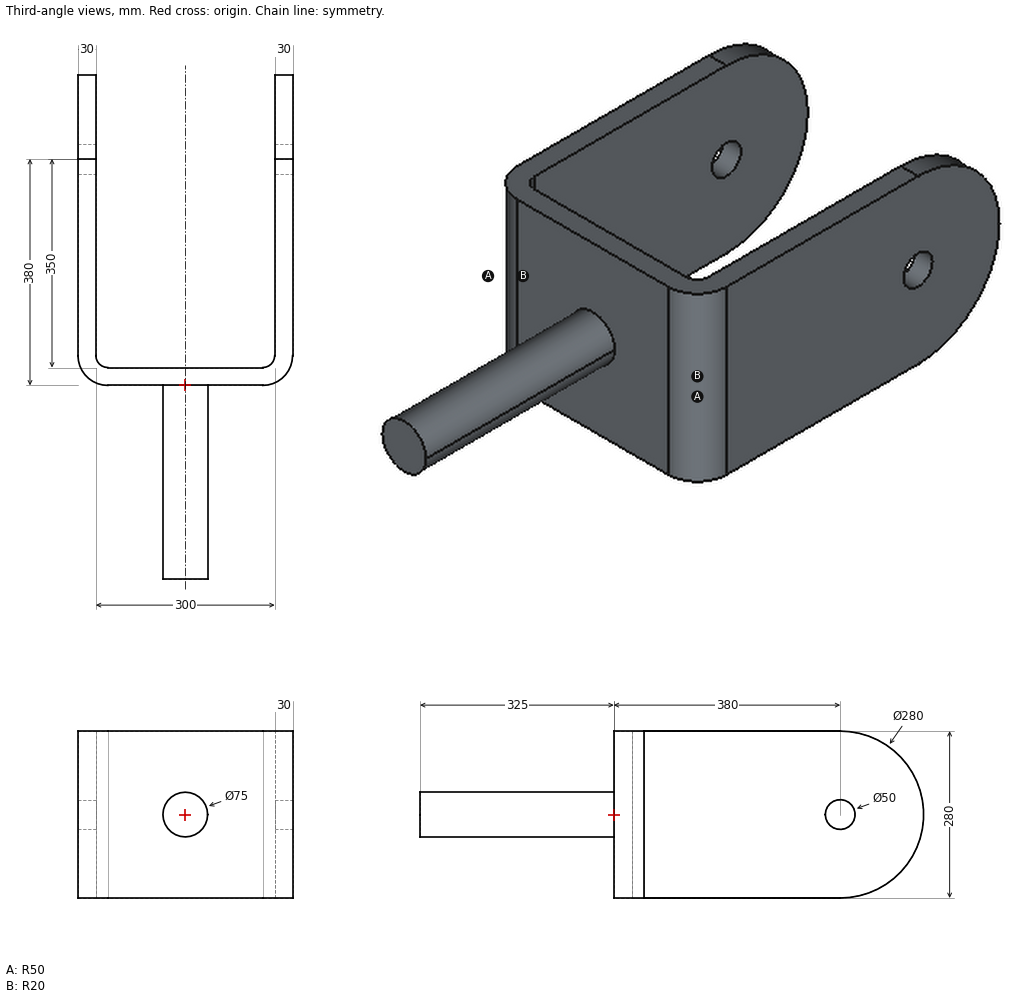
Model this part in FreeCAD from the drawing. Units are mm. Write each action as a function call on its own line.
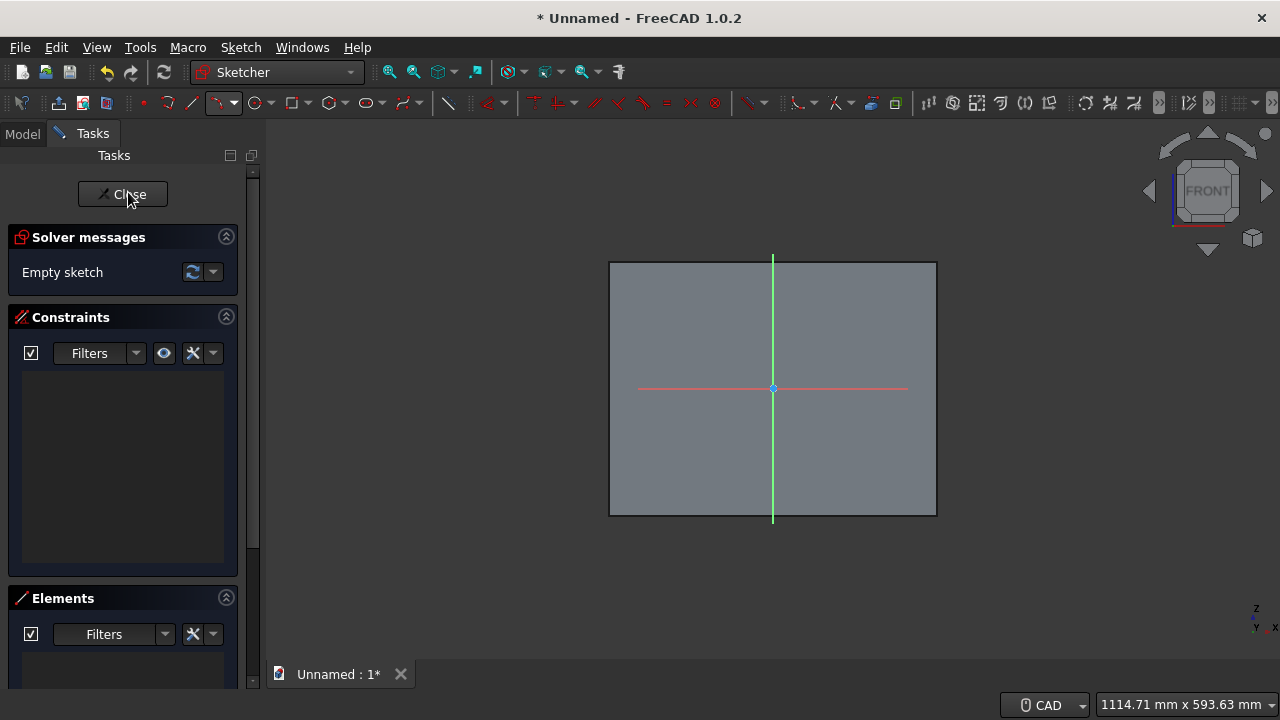
scroll(790, 389, up, 8)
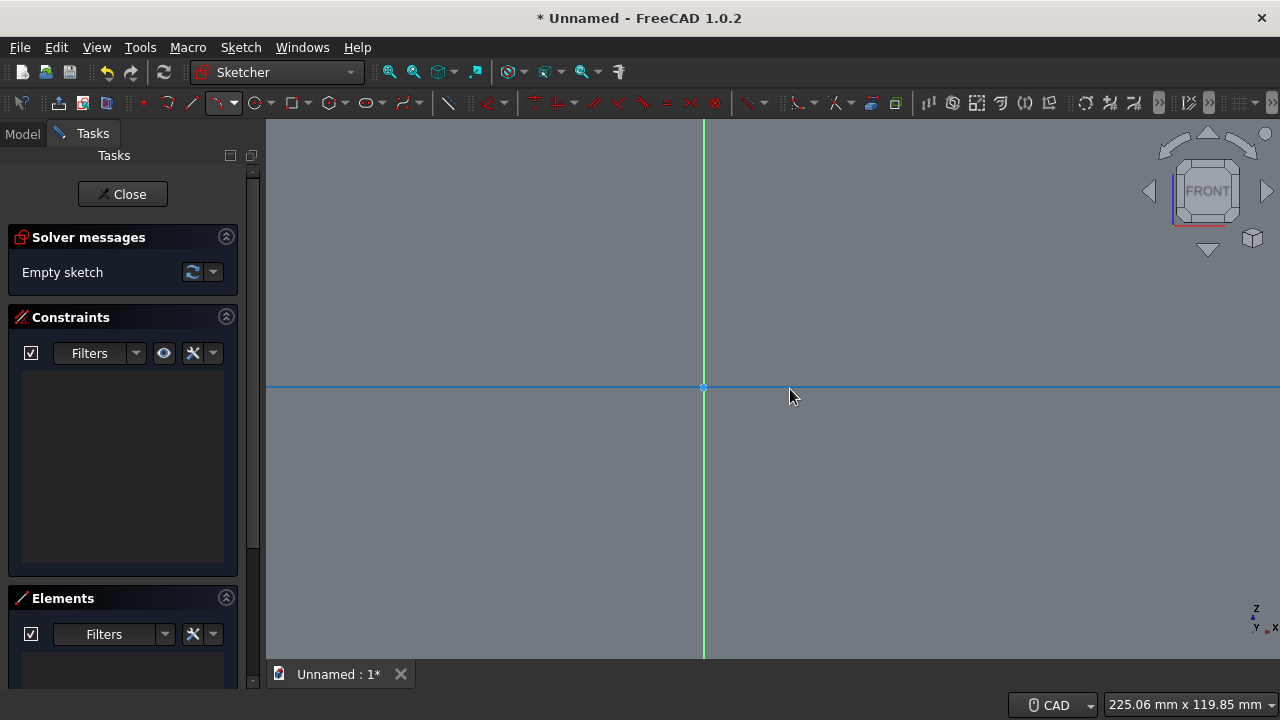
click(256, 104)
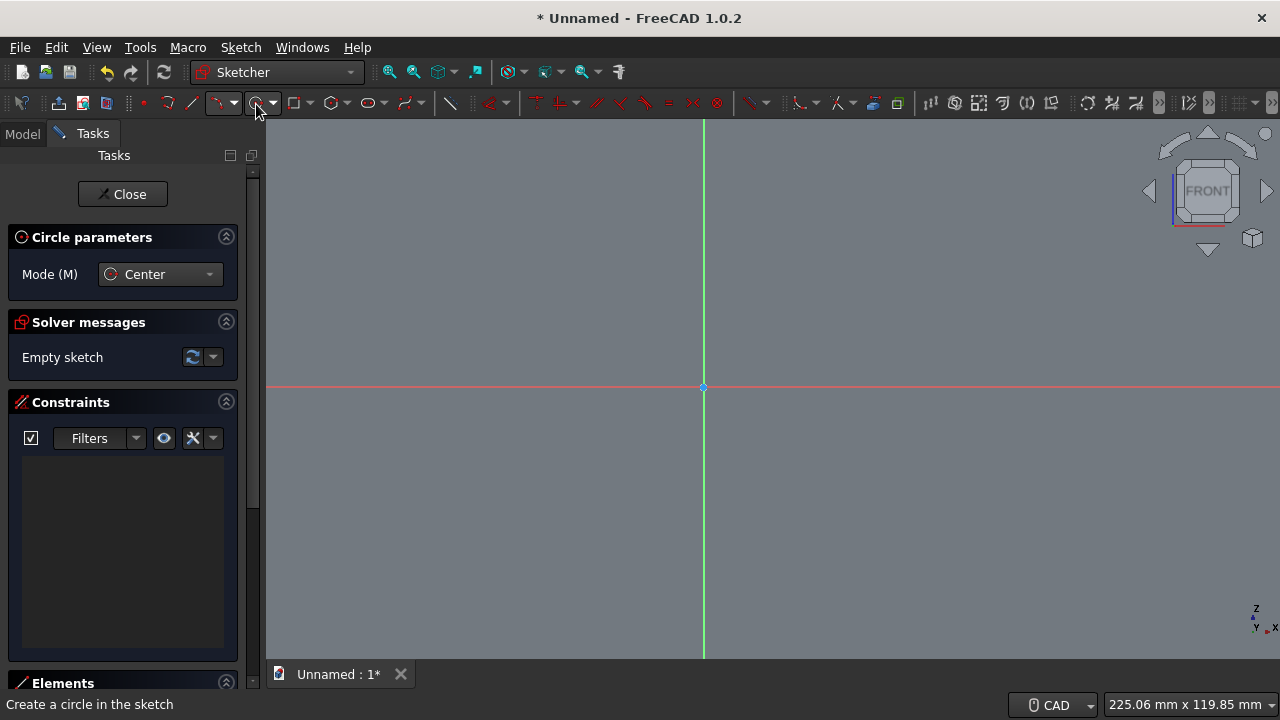
click(704, 387)
move(823, 268)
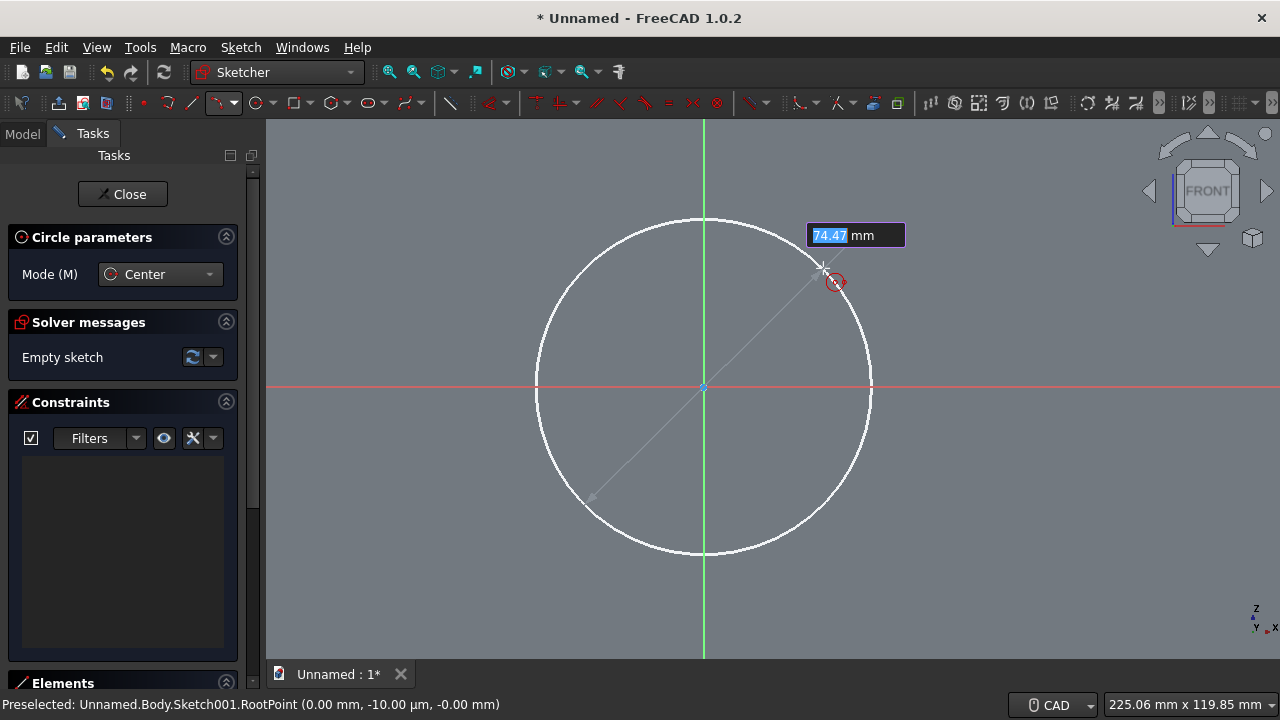
text(75)
key(Return)
key(Escape)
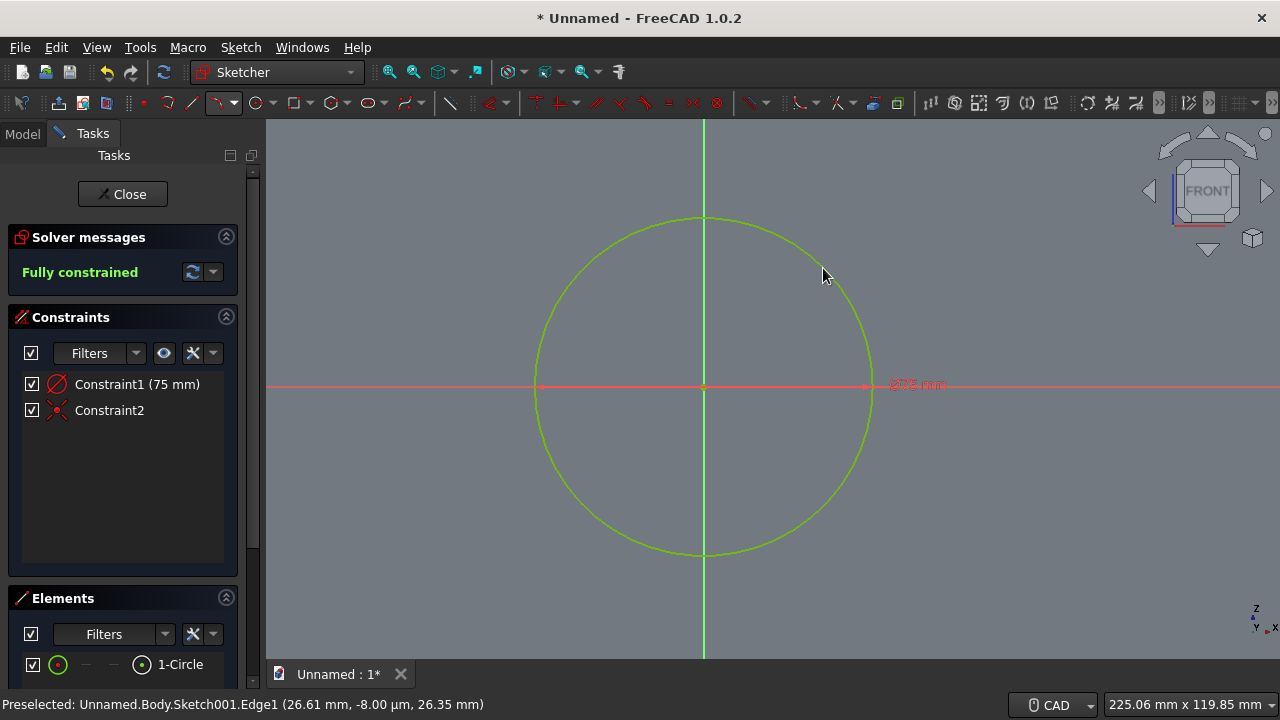
click(123, 194)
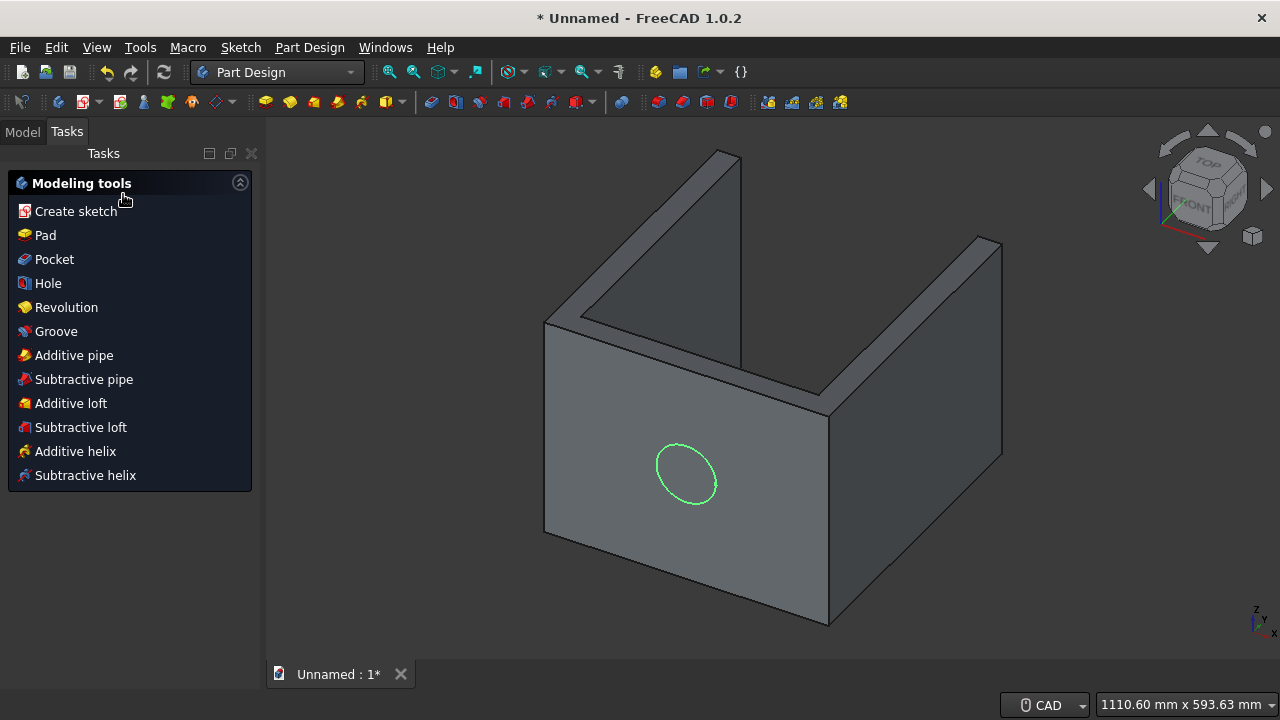
click(266, 102)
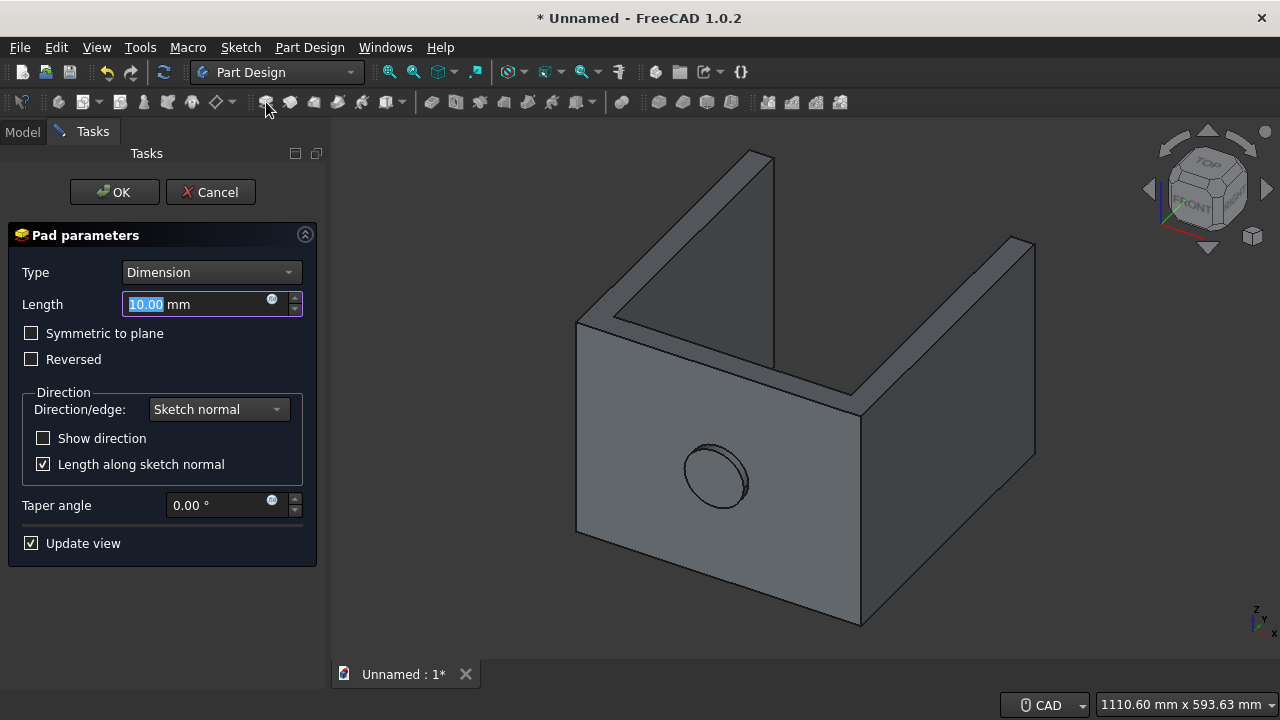
text(325)
key(Tab)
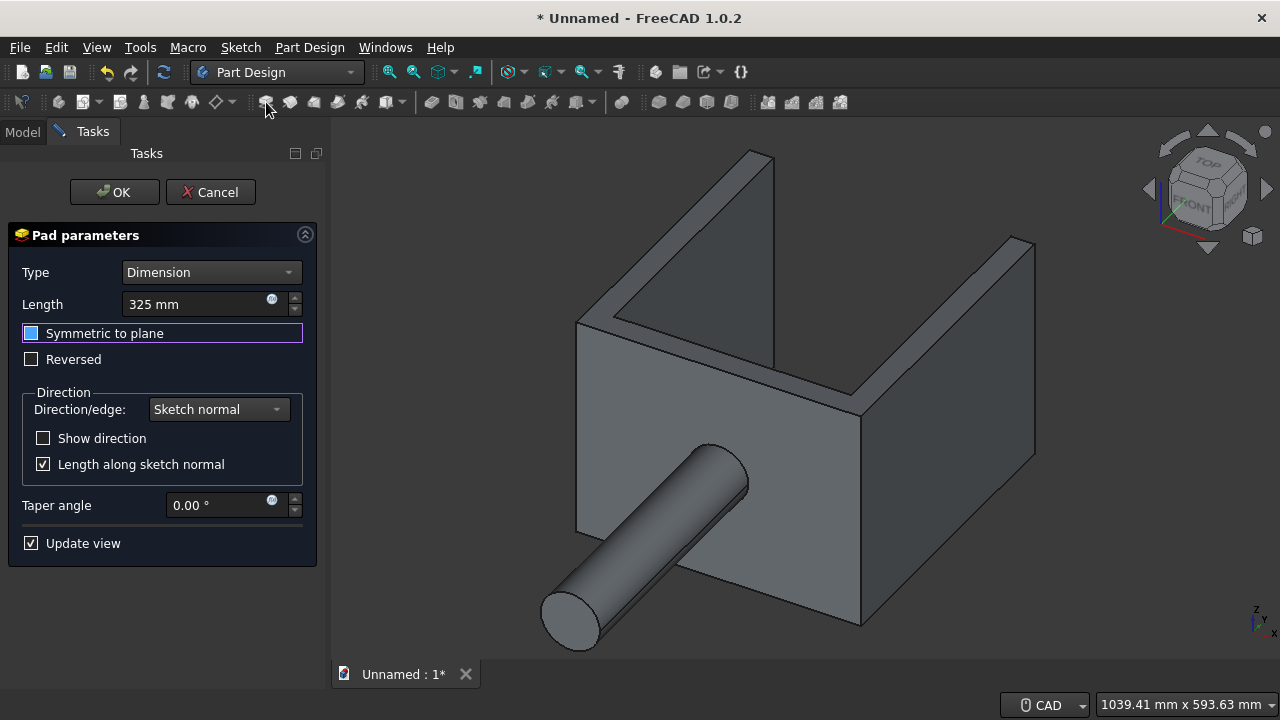
click(115, 192)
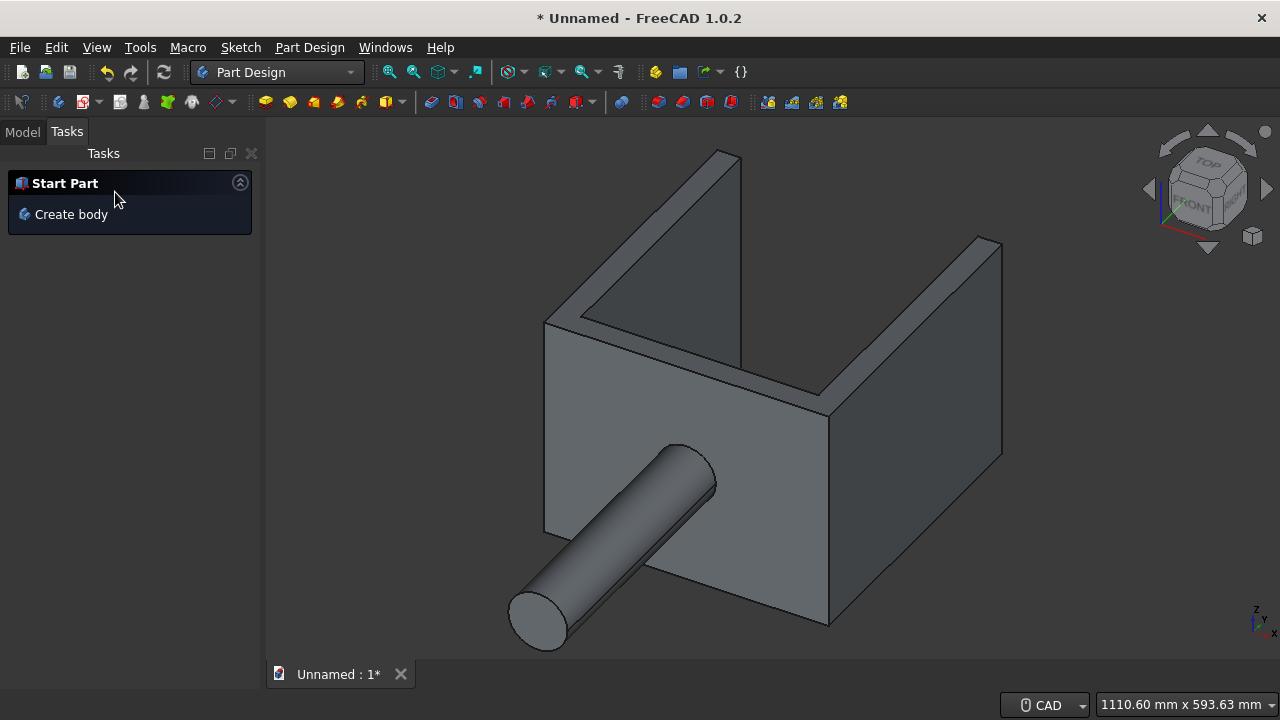
click(390, 72)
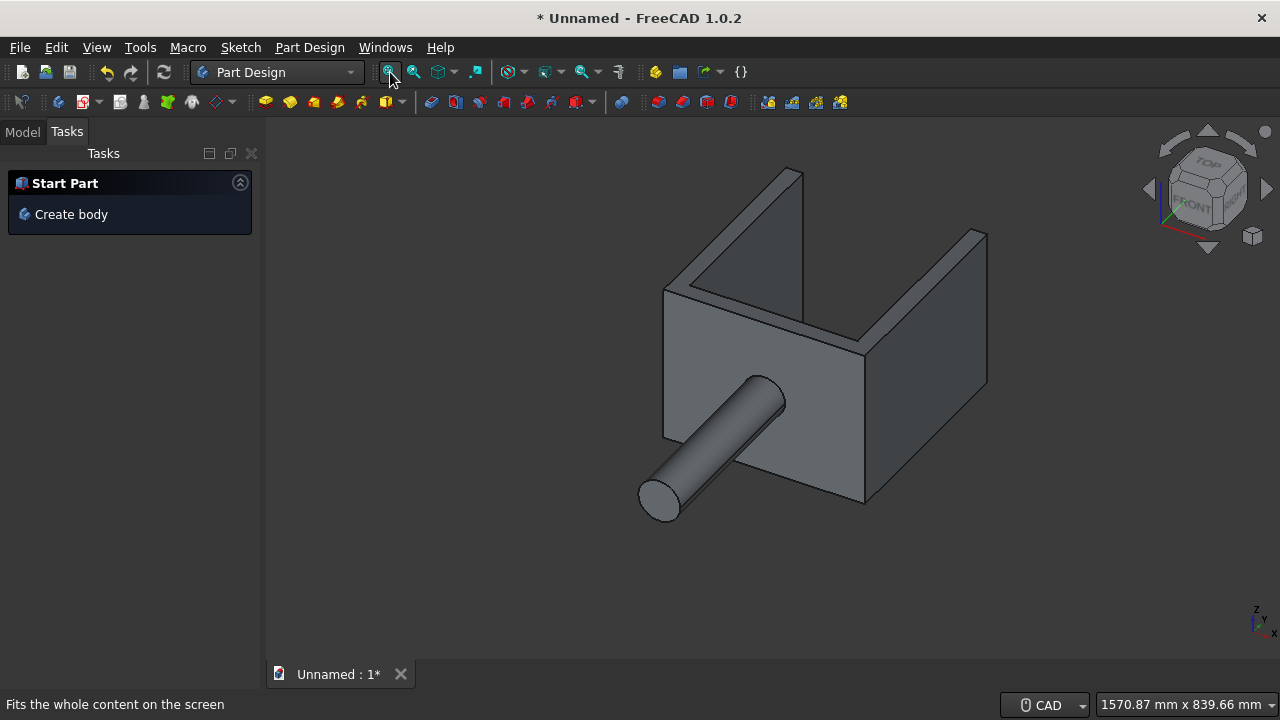
click(865, 429)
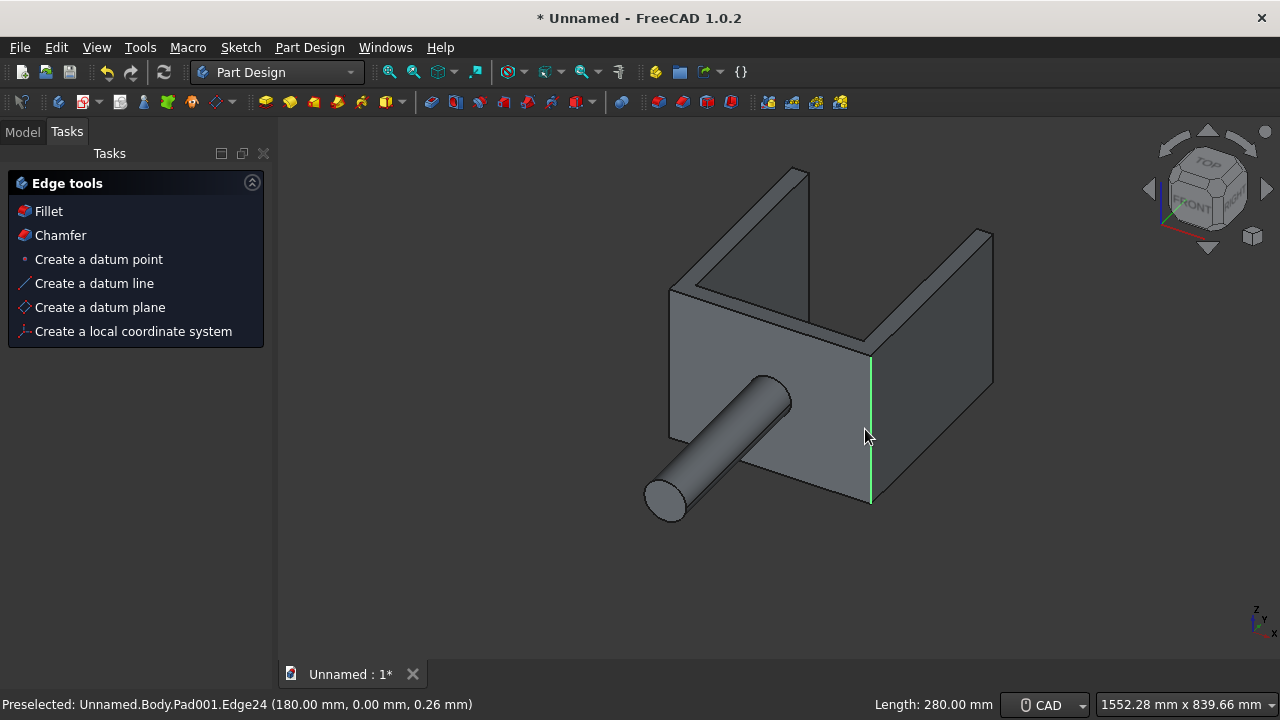
key(0)